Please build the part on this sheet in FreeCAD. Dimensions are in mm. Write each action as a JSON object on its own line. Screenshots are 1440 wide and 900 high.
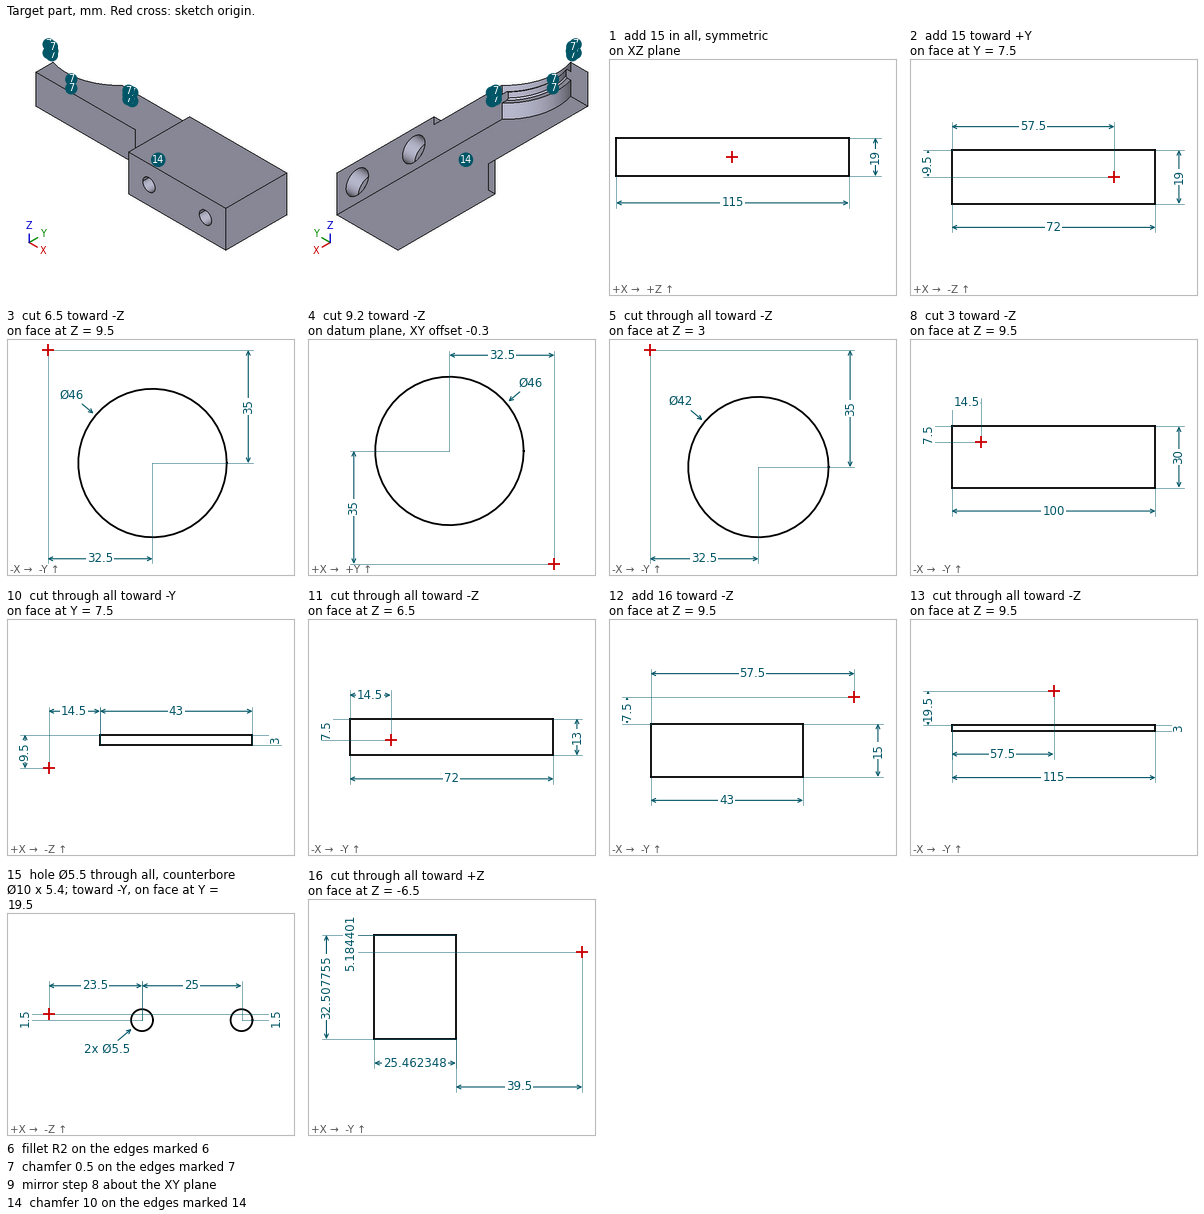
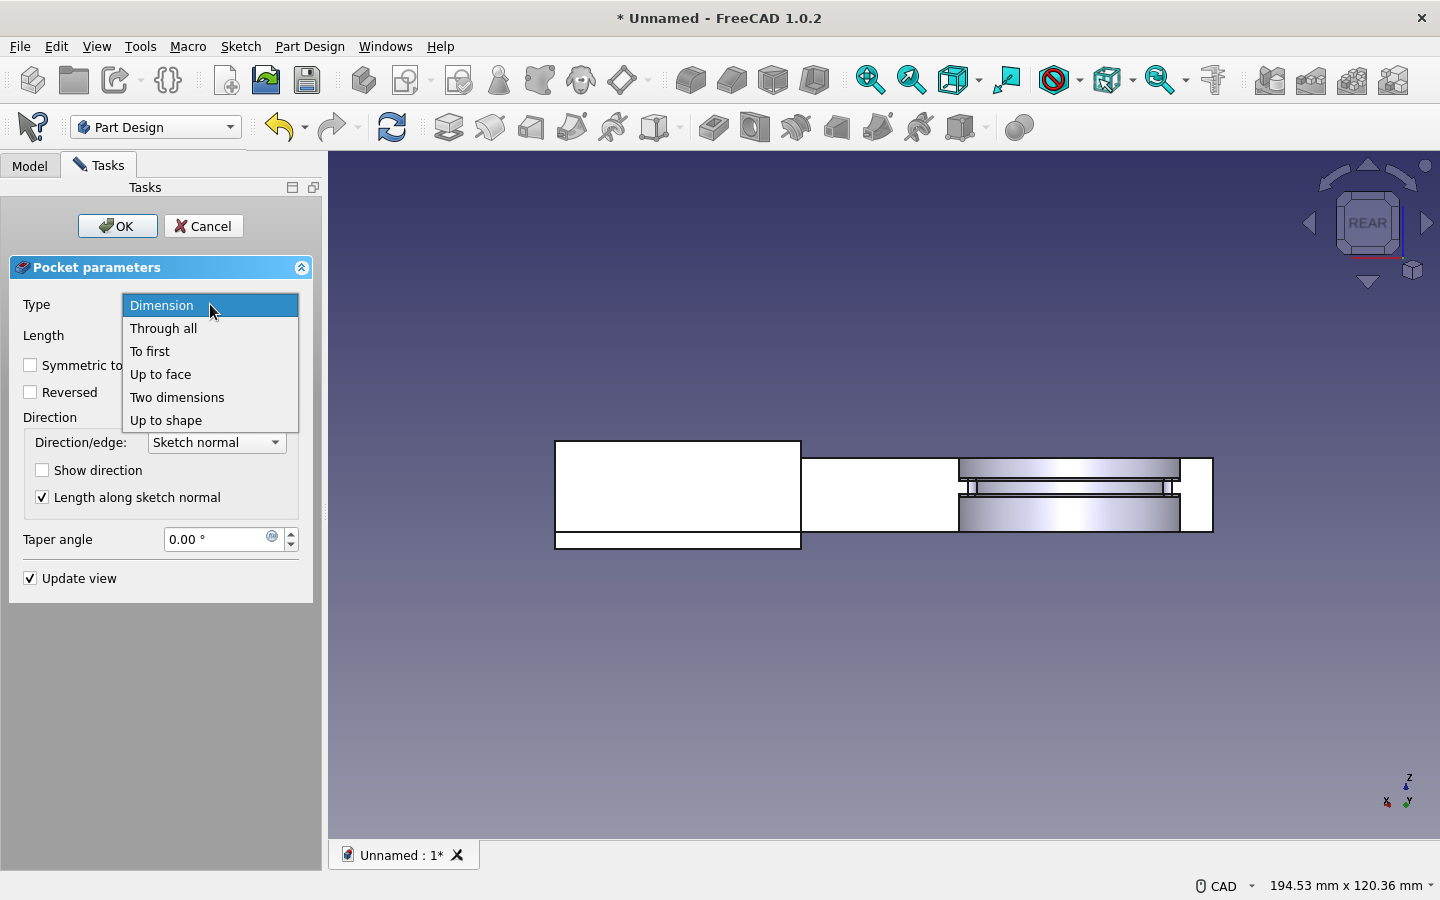
{"action": "left_click", "coordinate": [208, 328]}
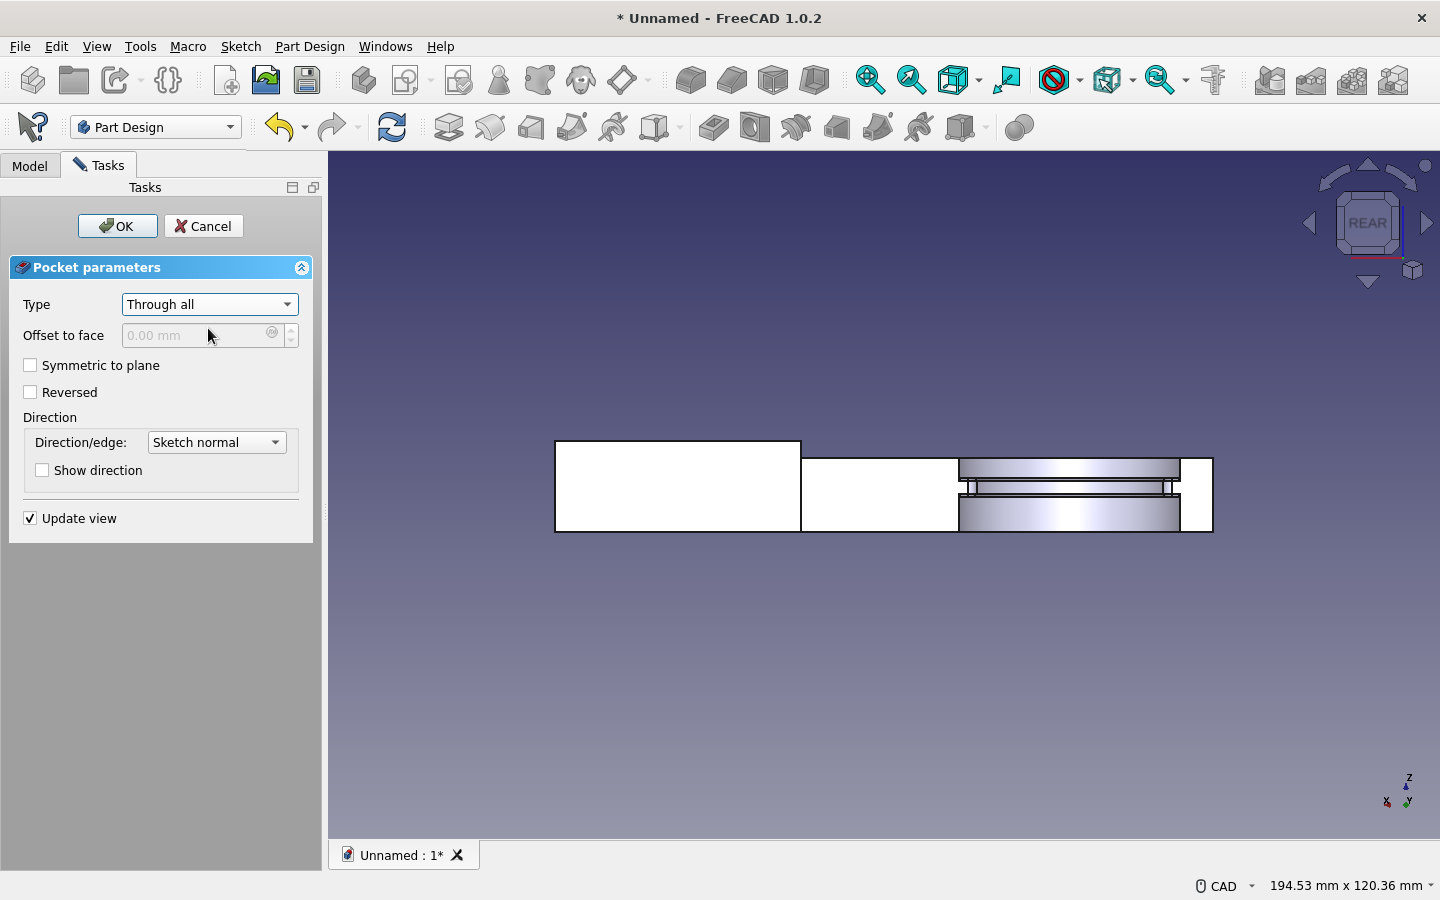
{"action": "left_click", "coordinate": [118, 226]}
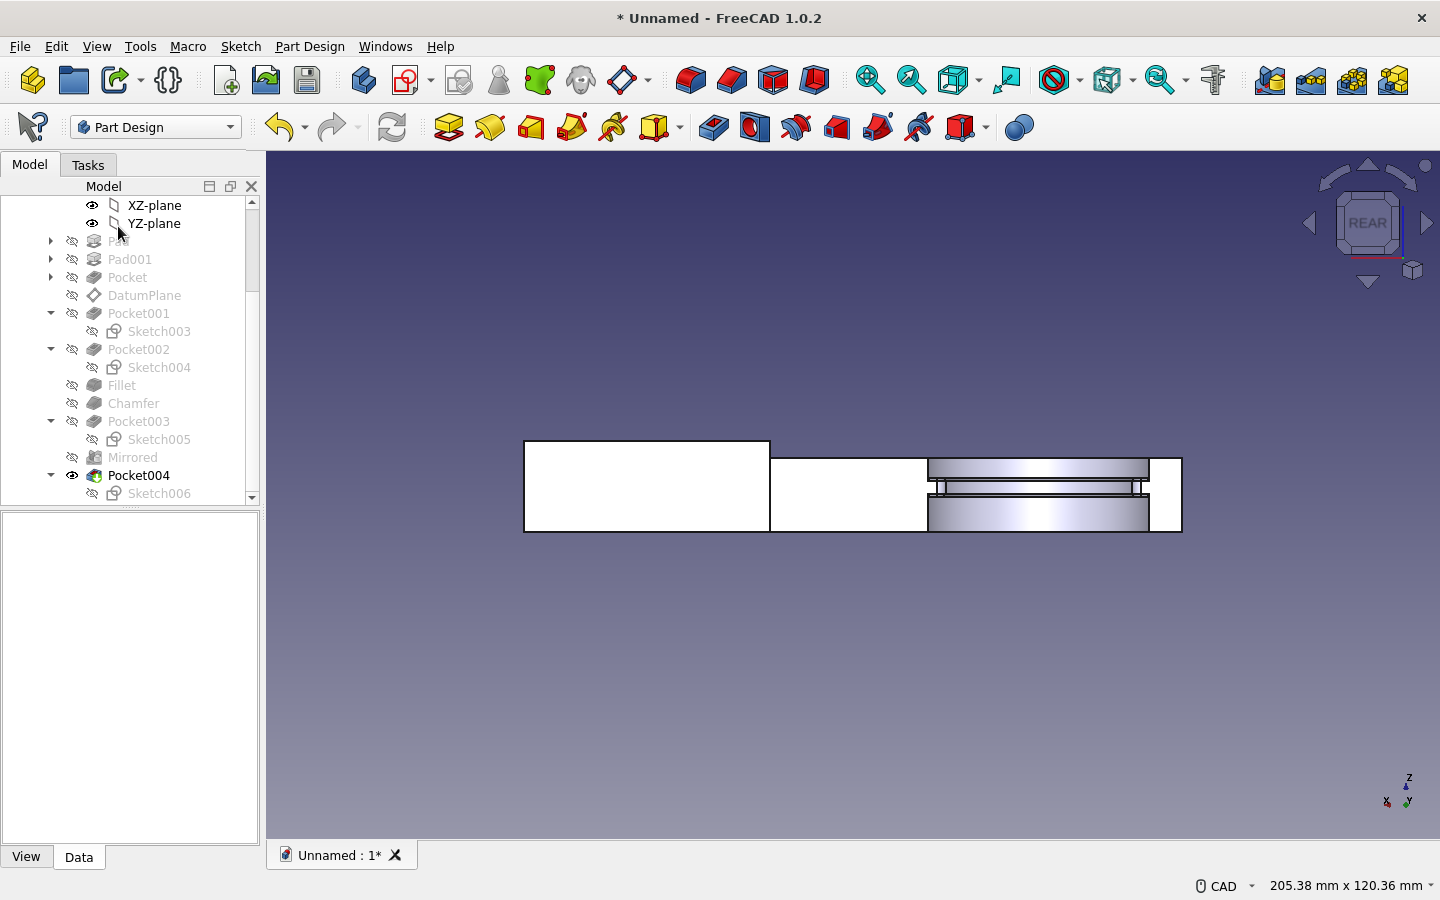
{"action": "key", "text": "0"}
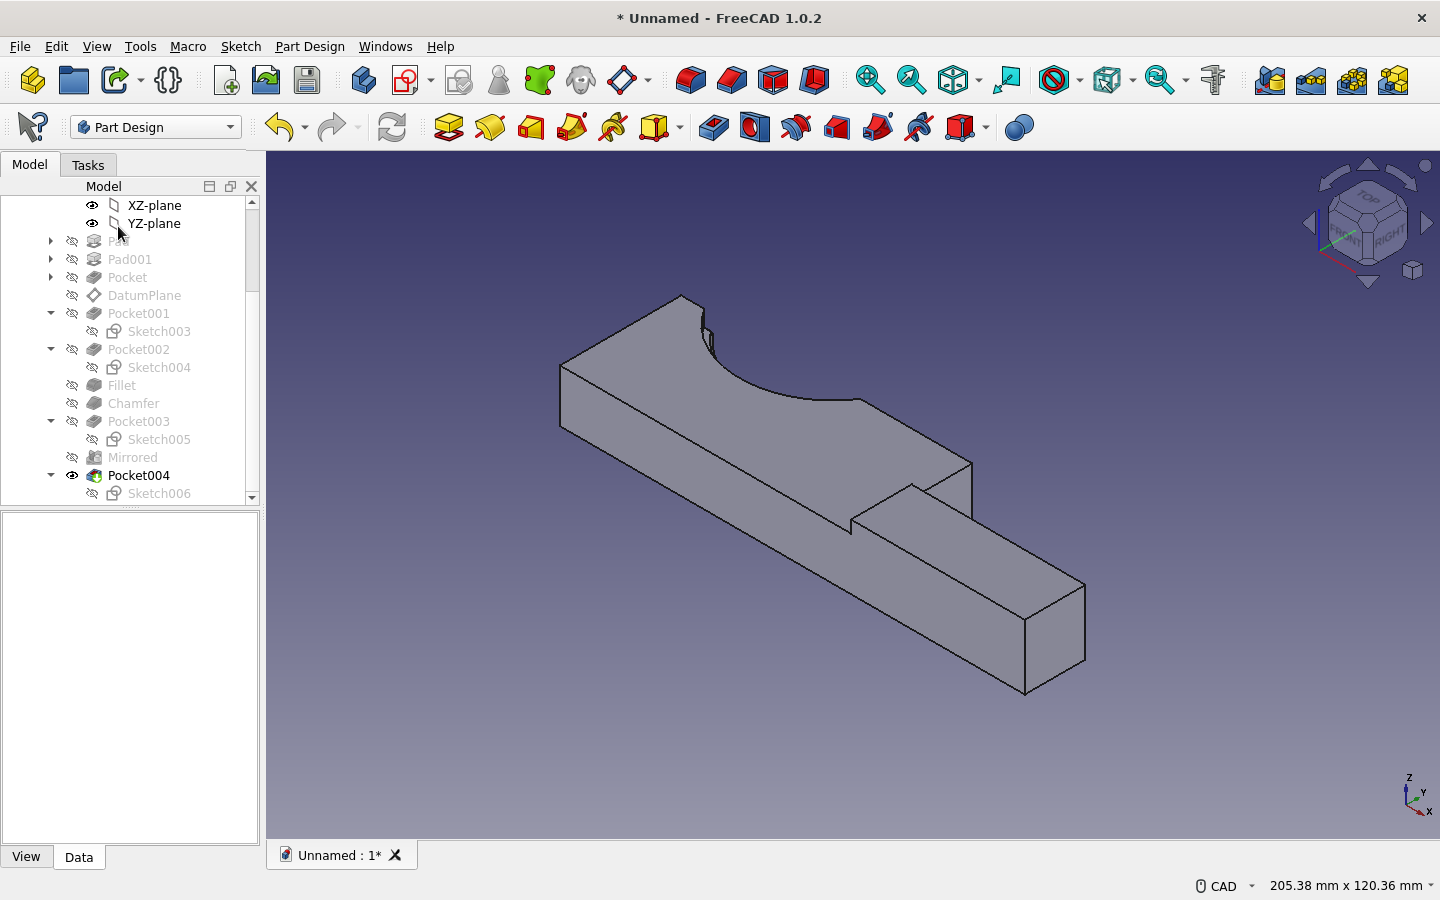
{"action": "left_click", "coordinate": [849, 461]}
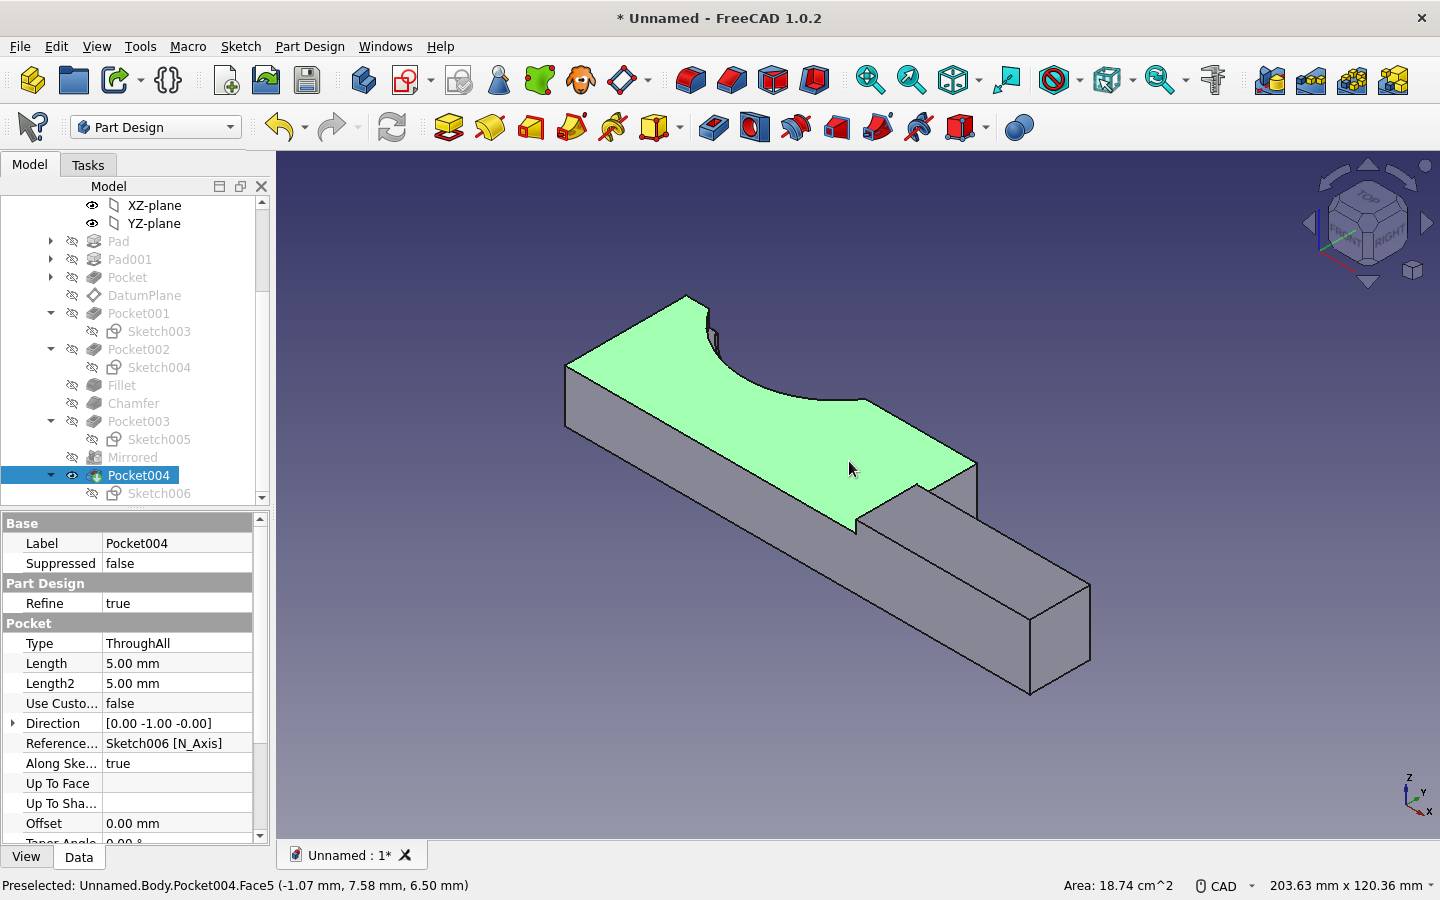
{"action": "left_click", "coordinate": [404, 80]}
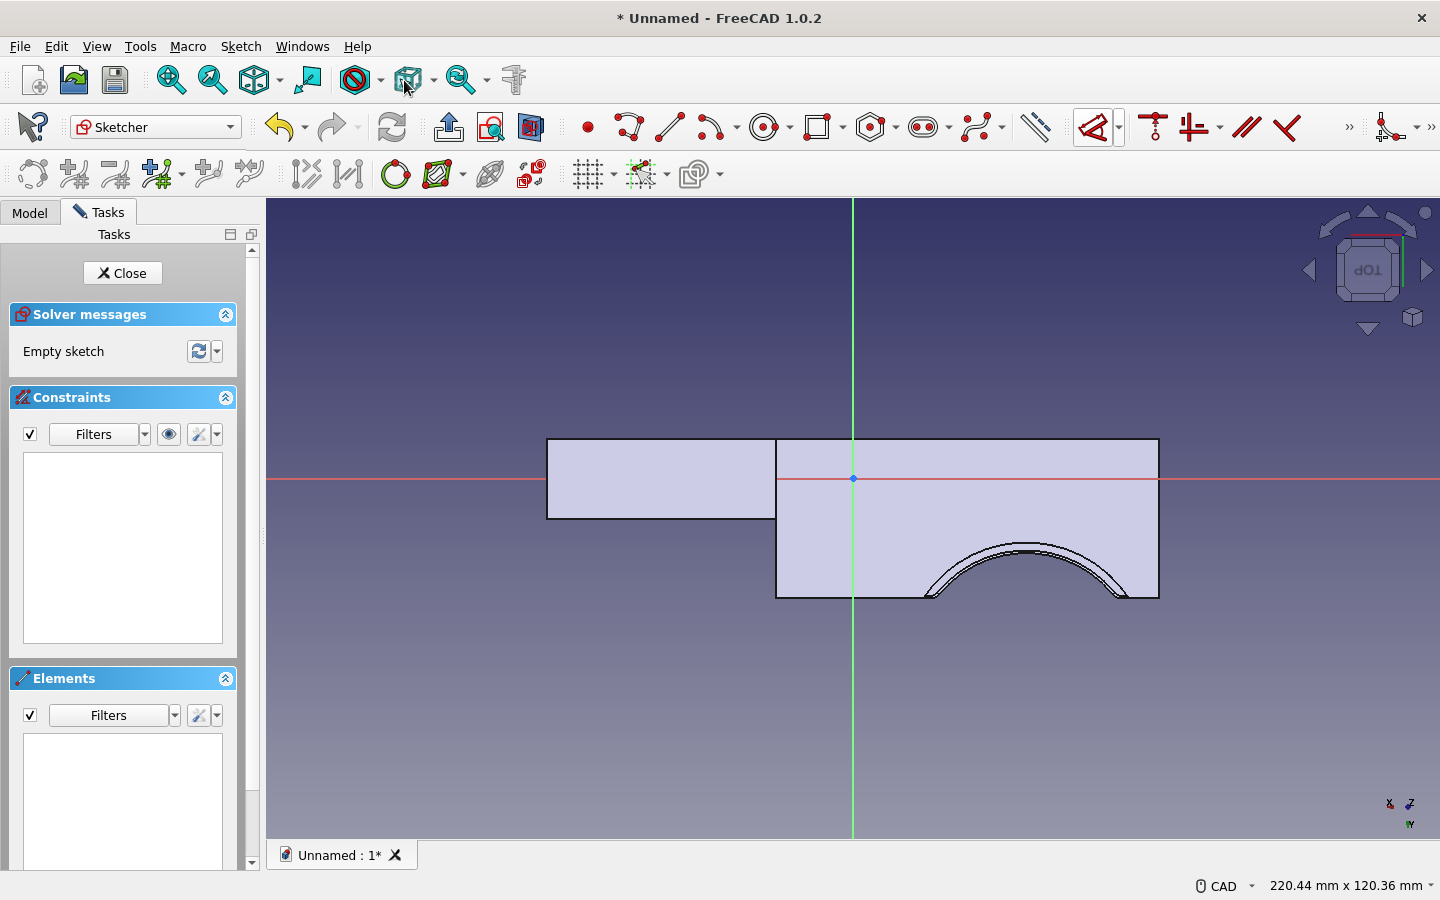
{"action": "left_click", "coordinate": [531, 128]}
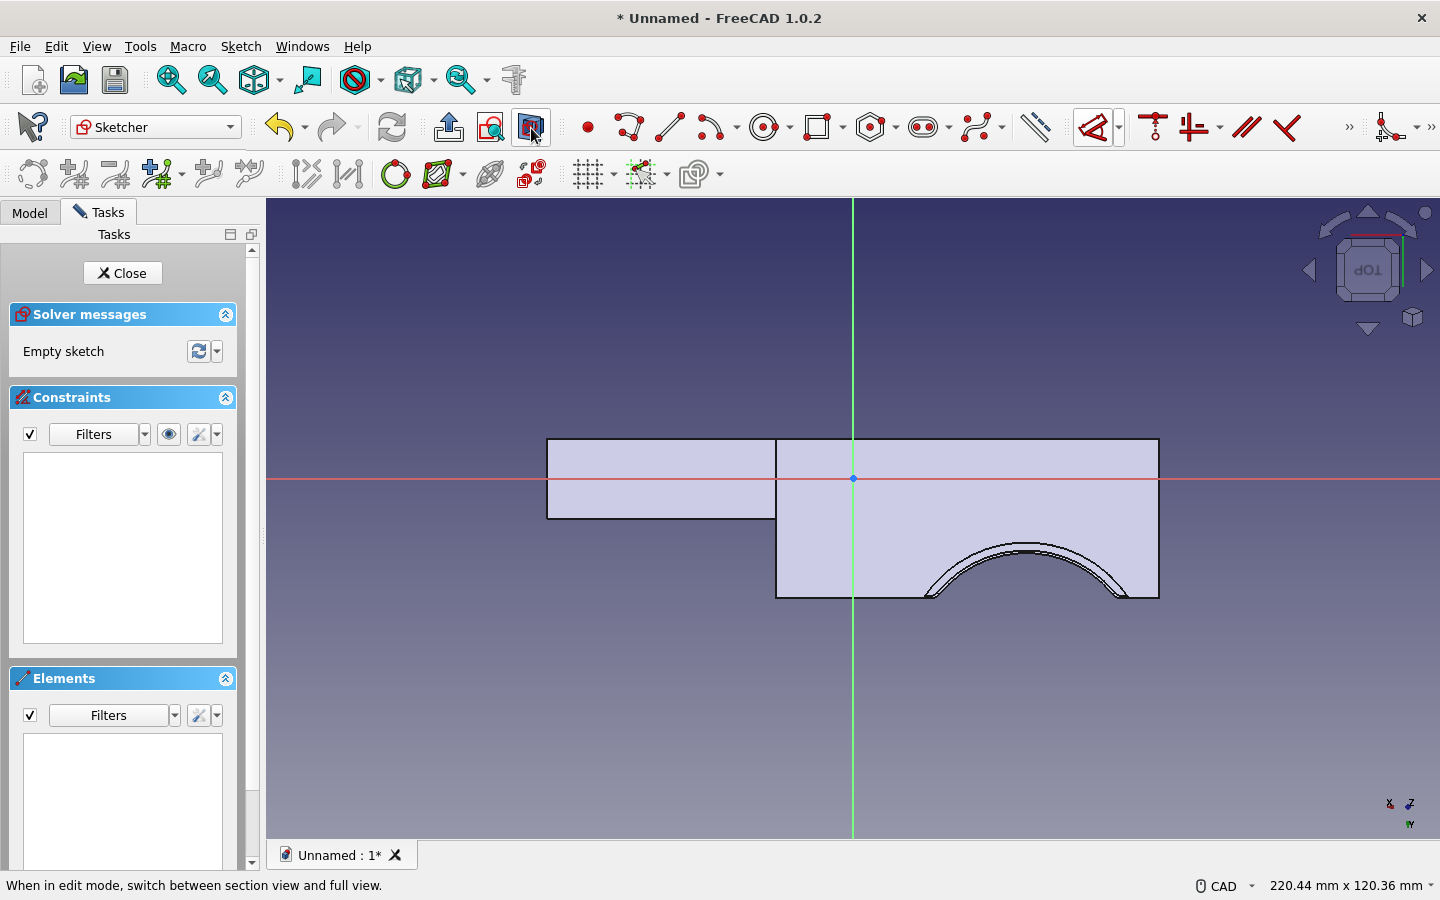
{"action": "scroll", "coordinate": [1190, 418], "scroll_direction": "up", "scroll_amount": 3}